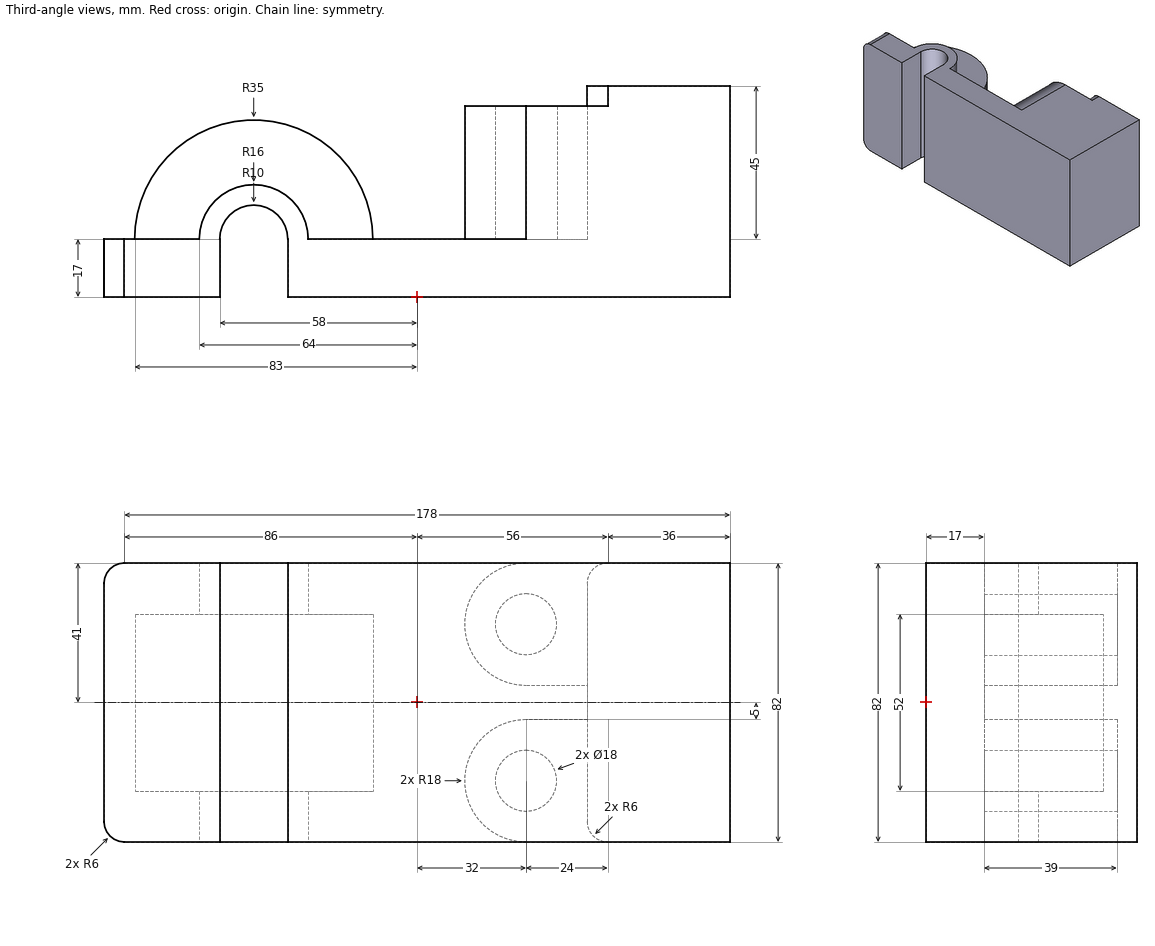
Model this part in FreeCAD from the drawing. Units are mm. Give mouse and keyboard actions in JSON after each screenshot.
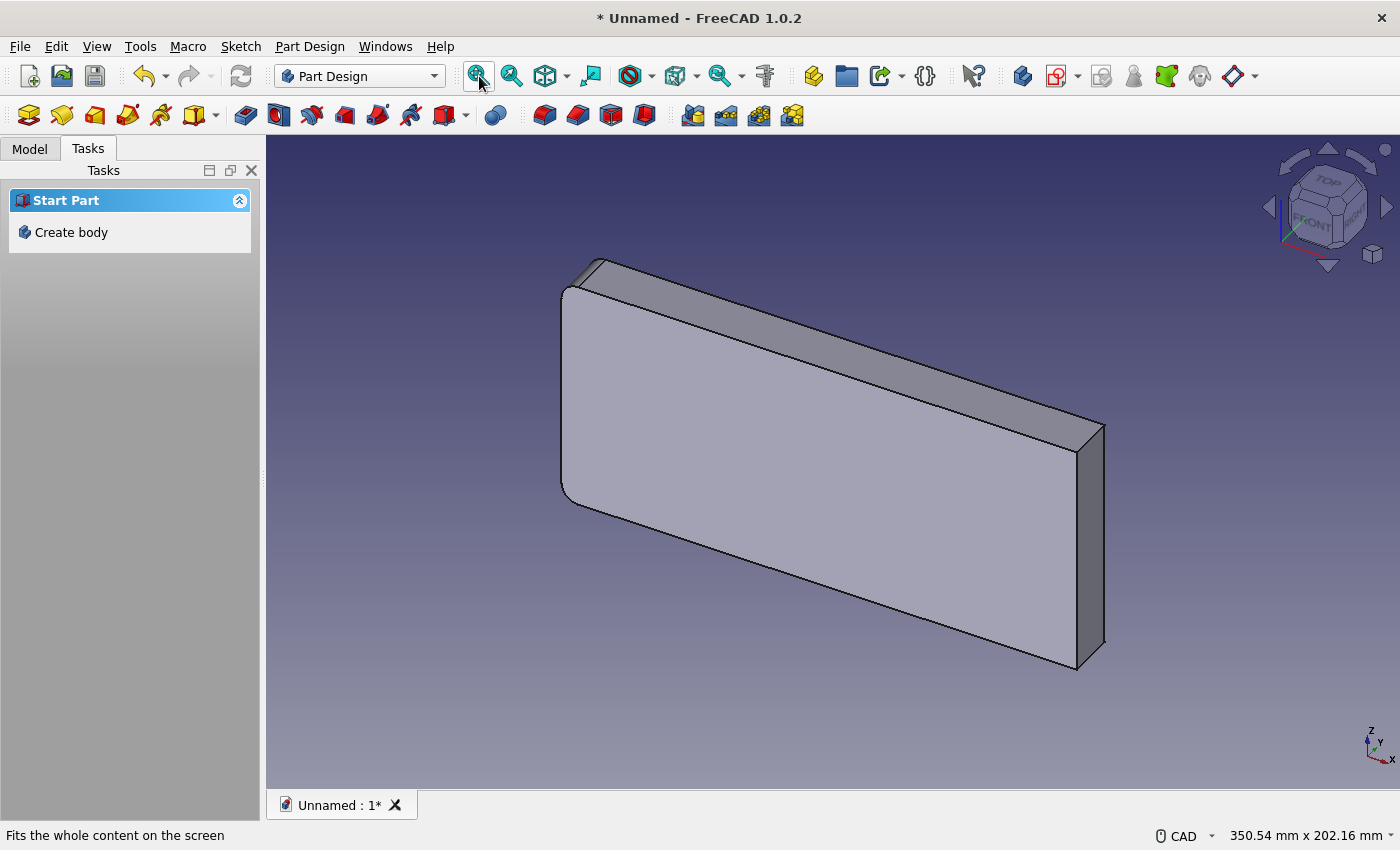
{"action": "key", "text": "4"}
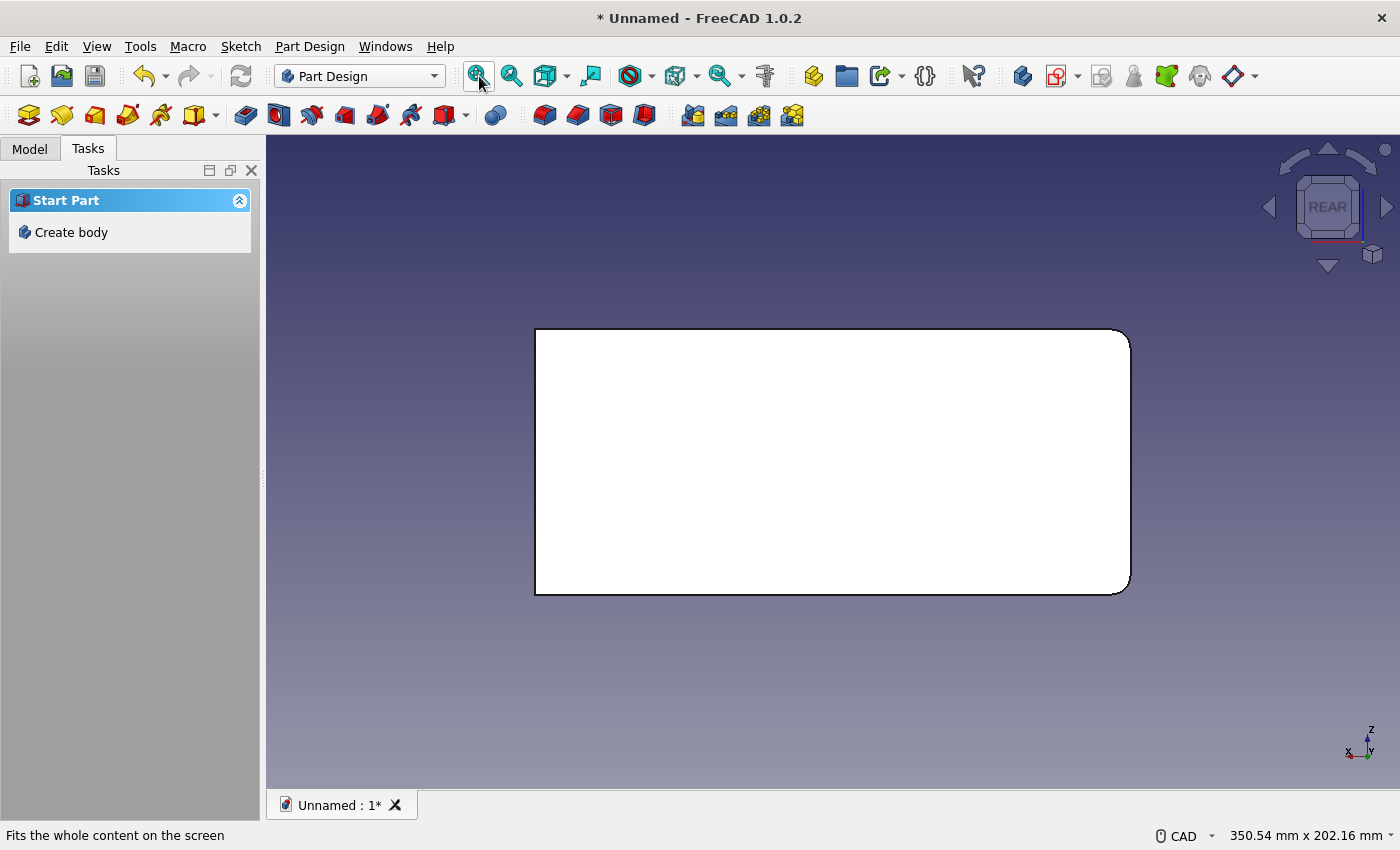
{"action": "left_click", "coordinate": [748, 461]}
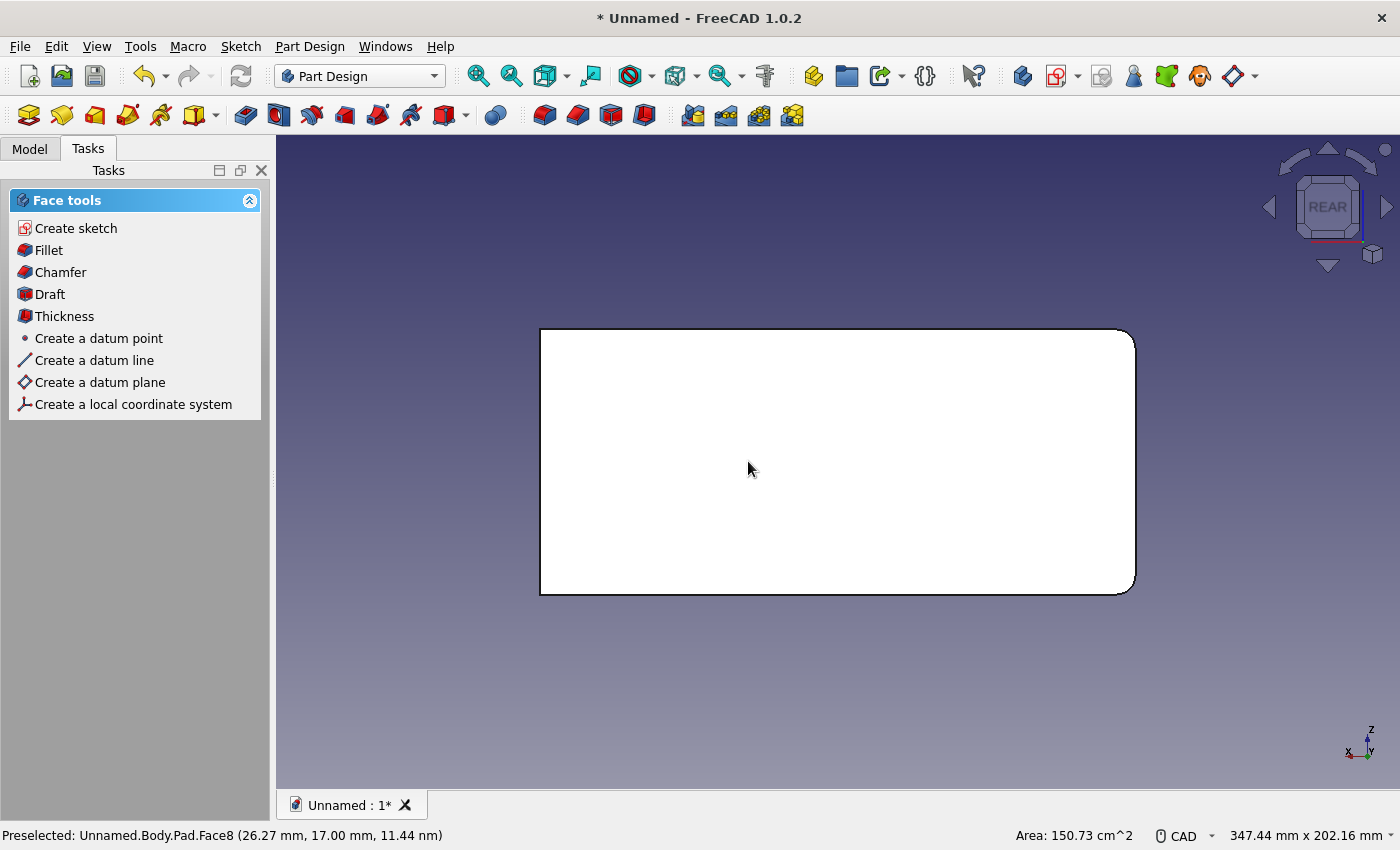
{"action": "left_click", "coordinate": [1056, 76]}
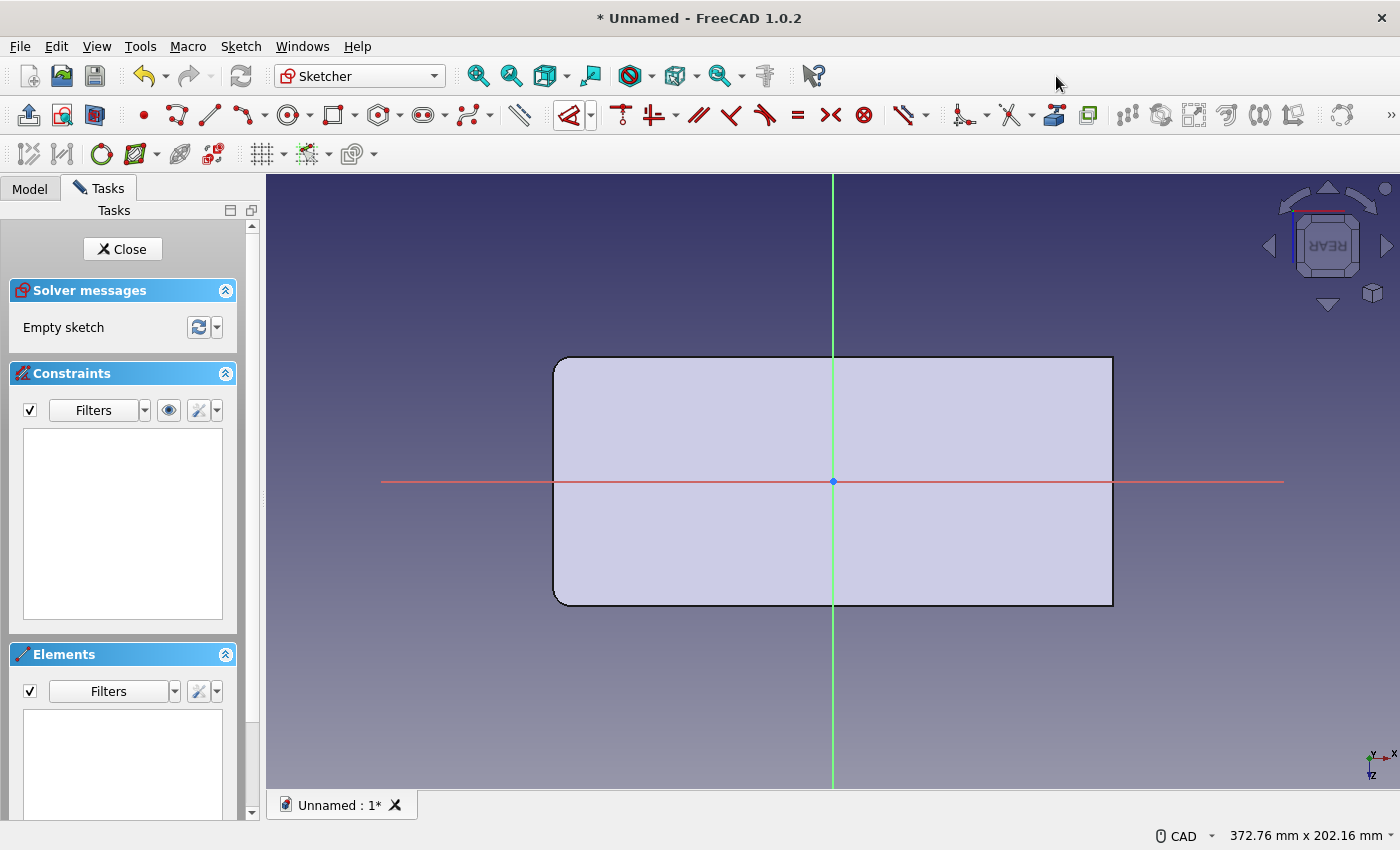
{"action": "scroll", "coordinate": [1235, 481], "scroll_direction": "up", "scroll_amount": 2}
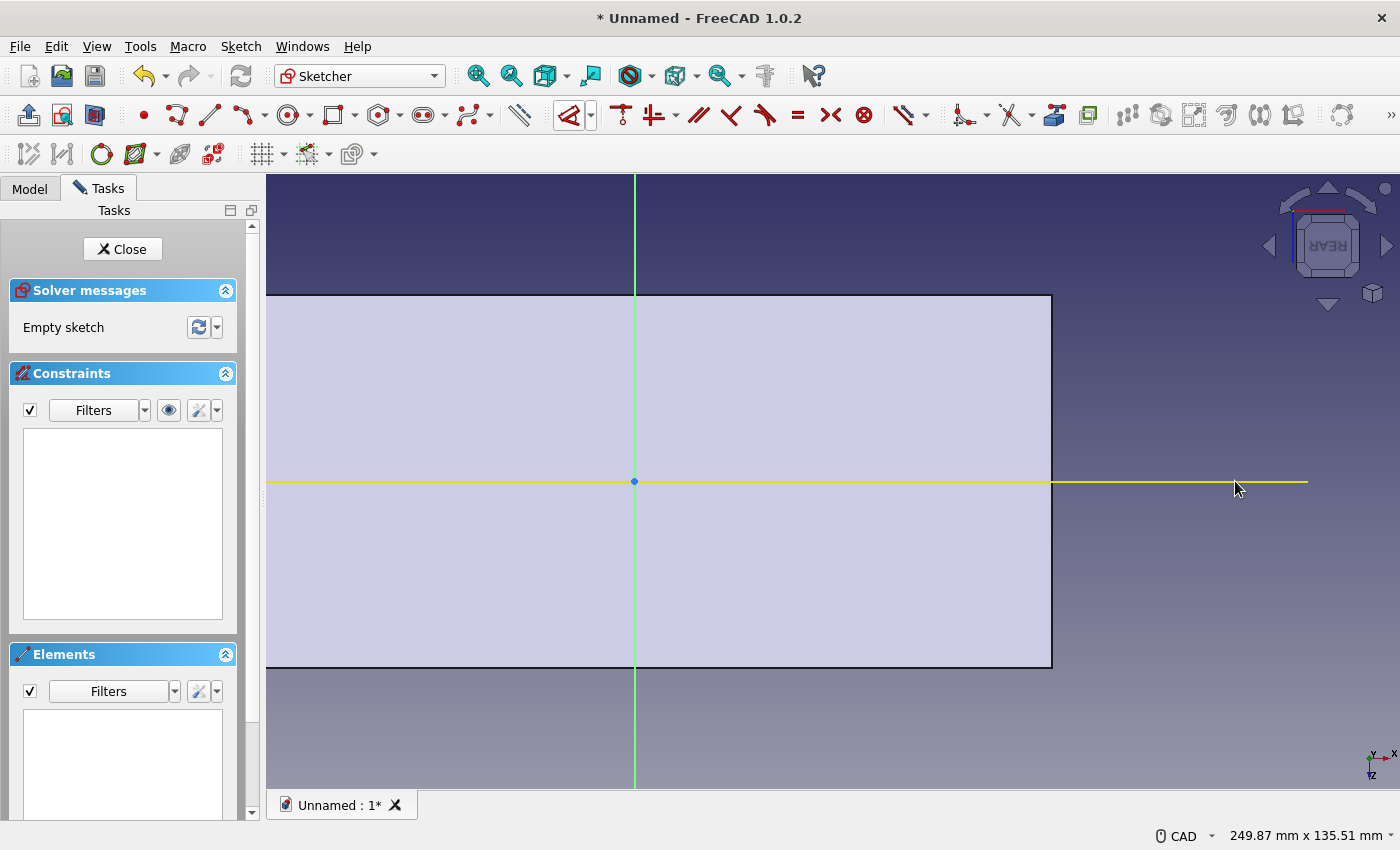
{"action": "left_click", "coordinate": [177, 116]}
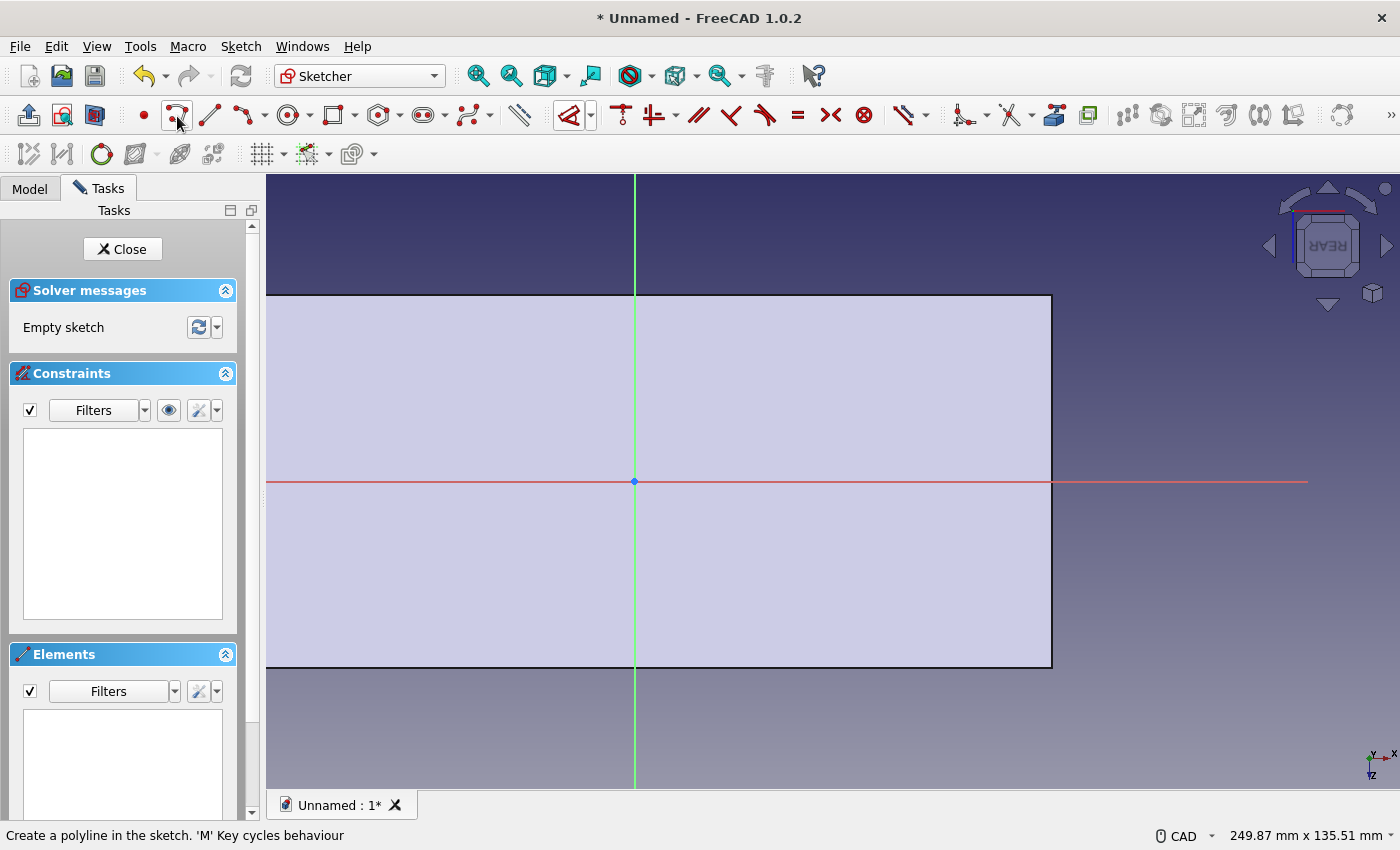
{"action": "left_click", "coordinate": [889, 668]}
{"action": "left_click", "coordinate": [1052, 668]}
{"action": "left_click", "coordinate": [1052, 295]}
{"action": "left_click", "coordinate": [889, 295]}
{"action": "right_click", "coordinate": [889, 295]}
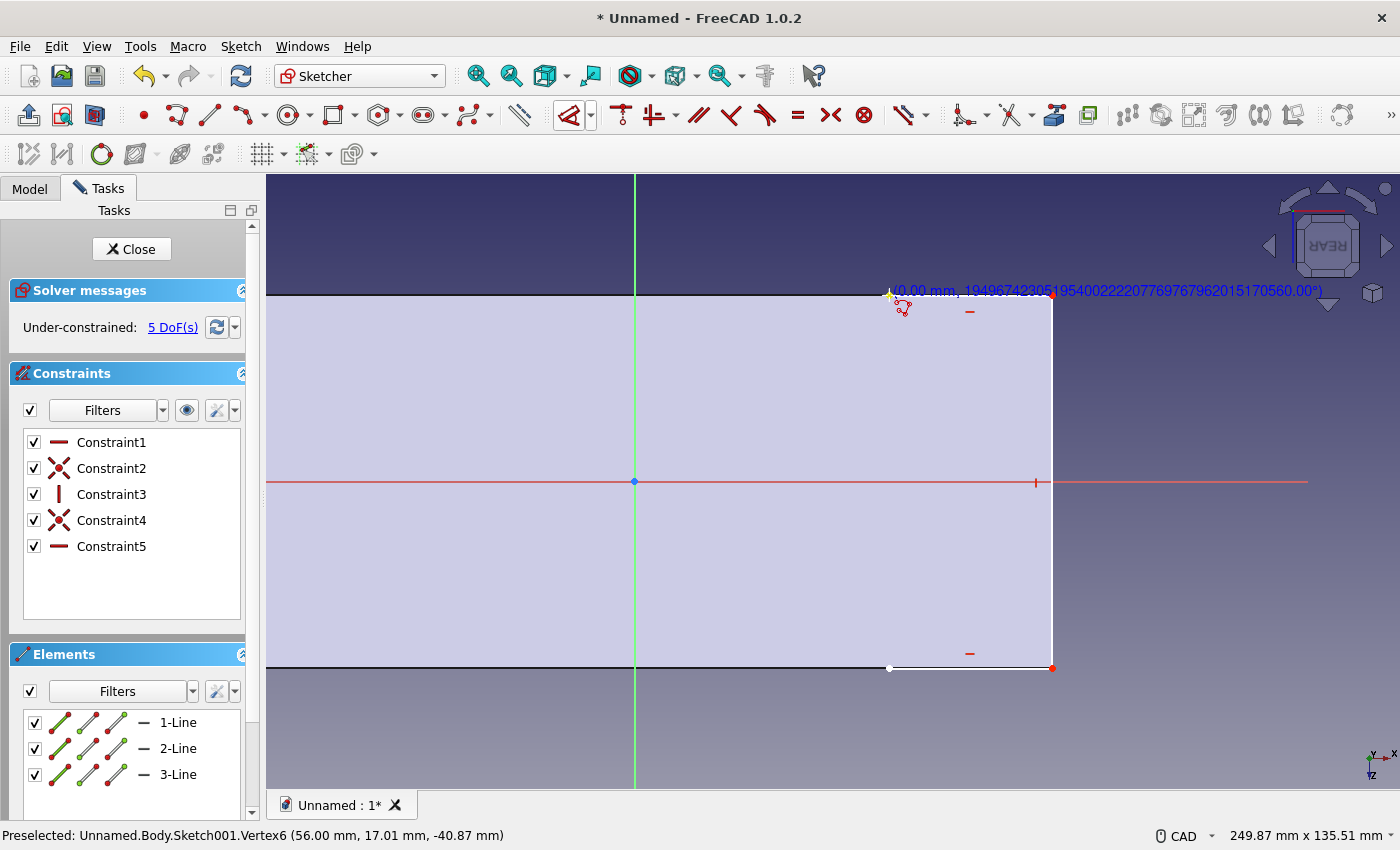
{"action": "left_click", "coordinate": [210, 116]}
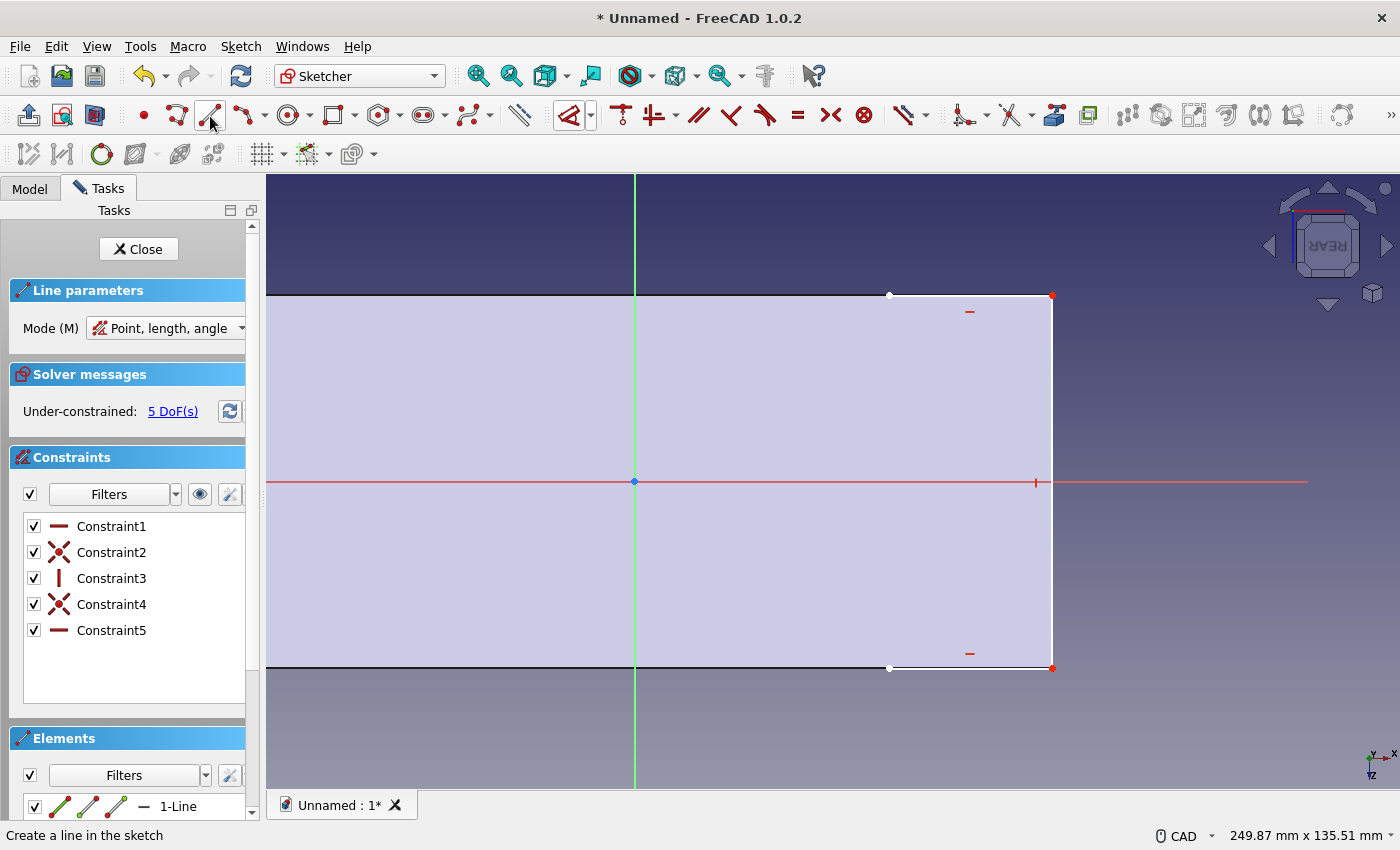
{"action": "left_click", "coordinate": [862, 323]}
{"action": "left_click", "coordinate": [862, 640]}